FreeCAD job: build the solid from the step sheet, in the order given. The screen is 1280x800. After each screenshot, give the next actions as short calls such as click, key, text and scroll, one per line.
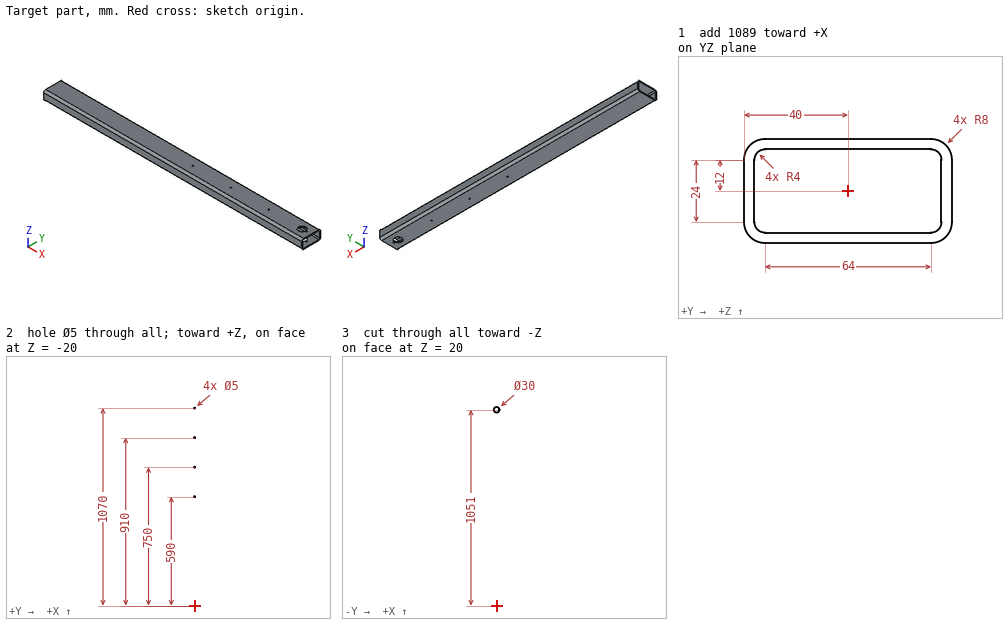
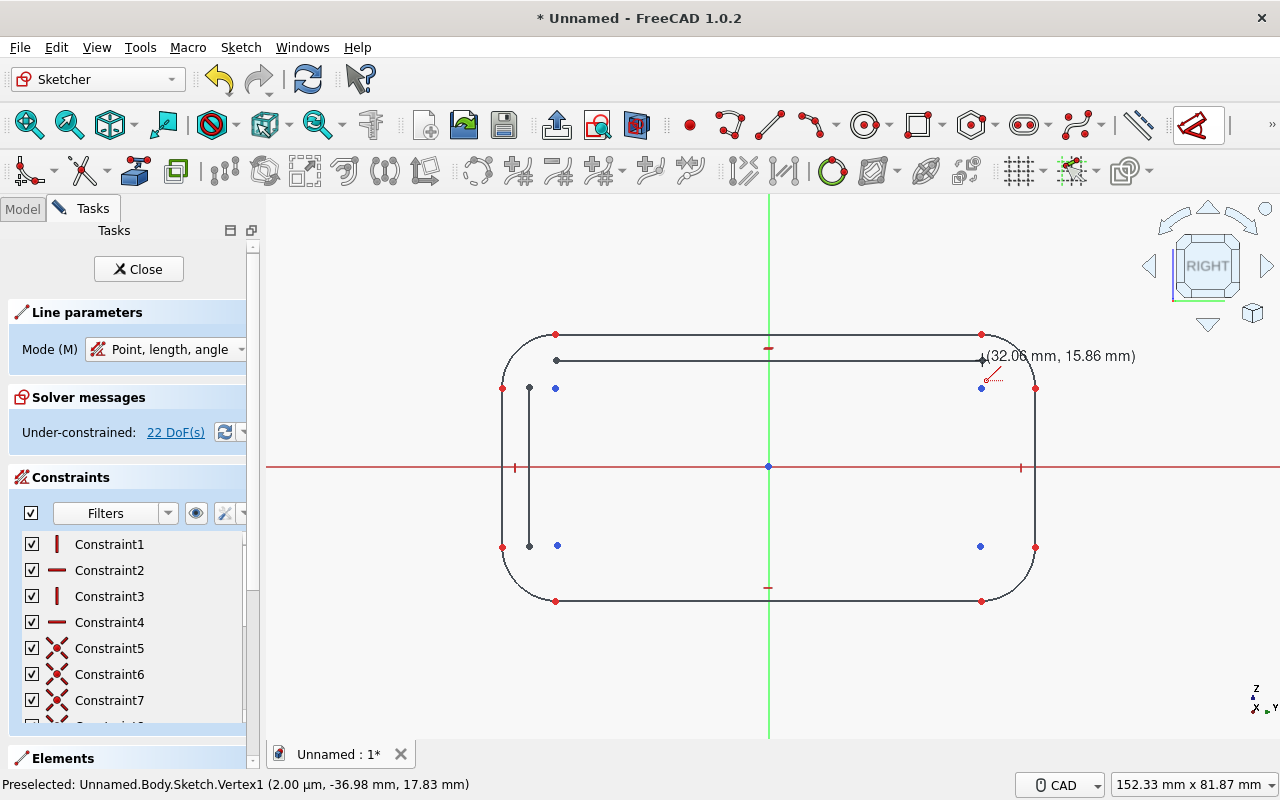
click(1008, 387)
click(1008, 546)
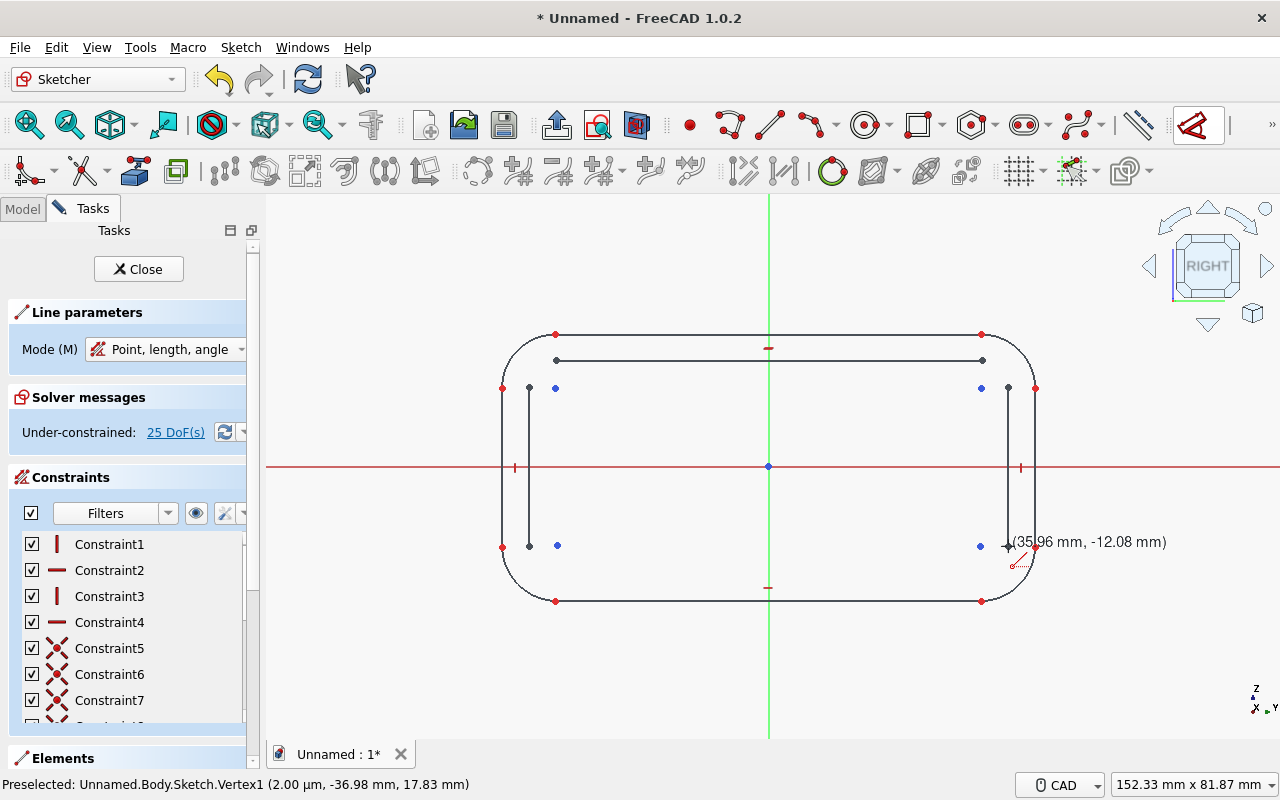
click(982, 573)
click(556, 573)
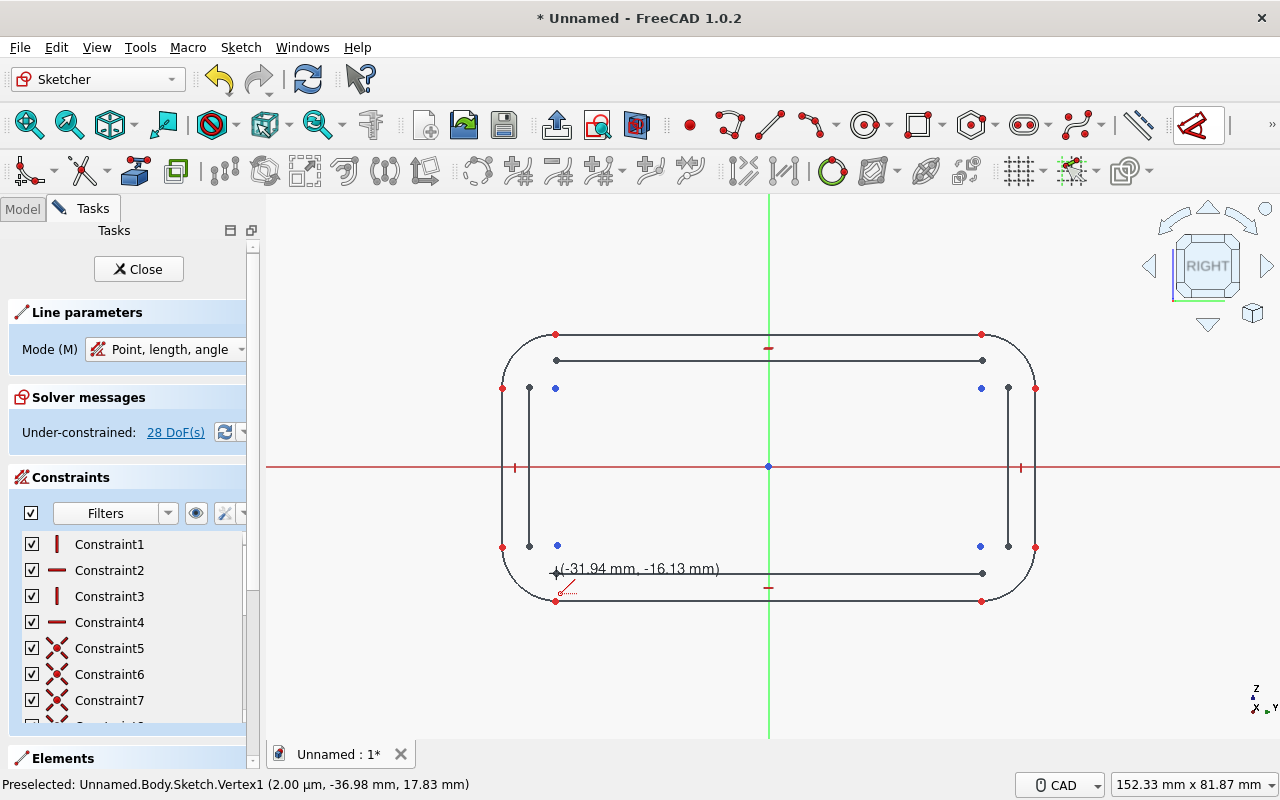
click(812, 126)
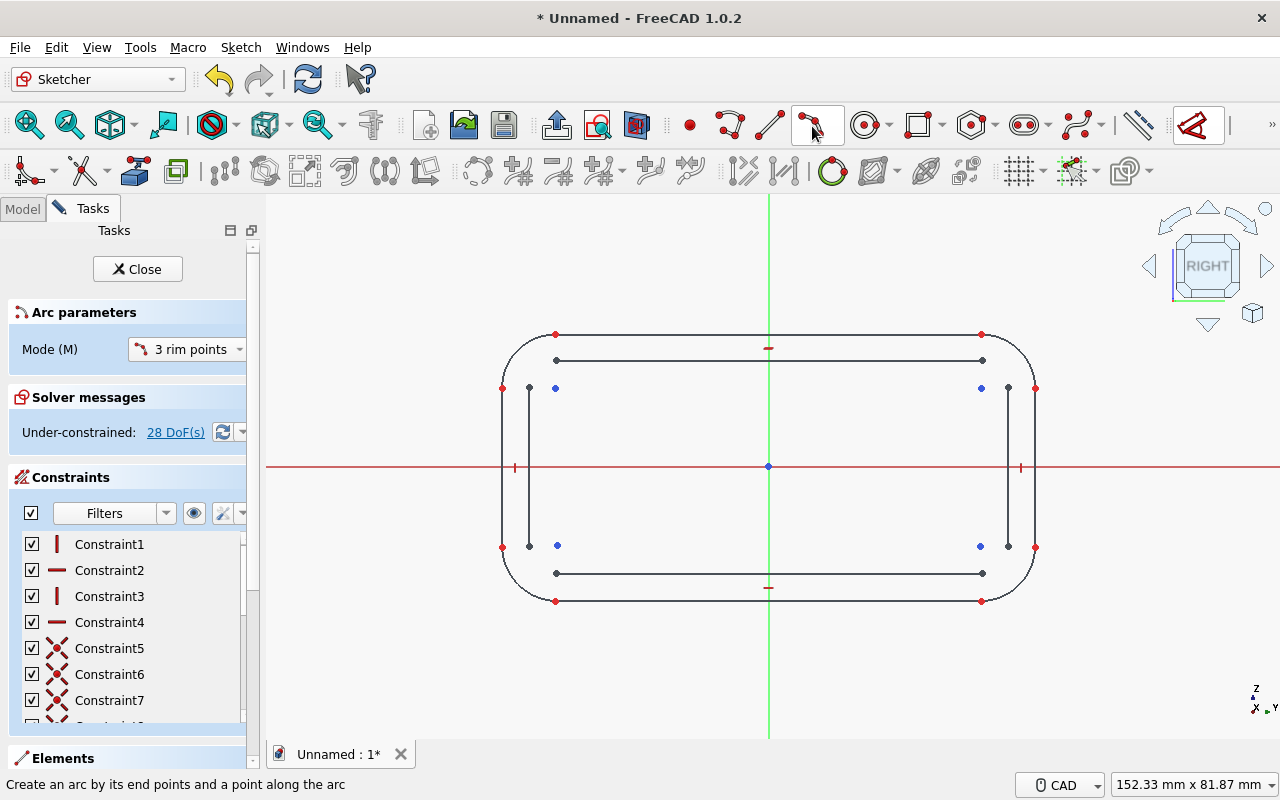
click(529, 388)
click(556, 361)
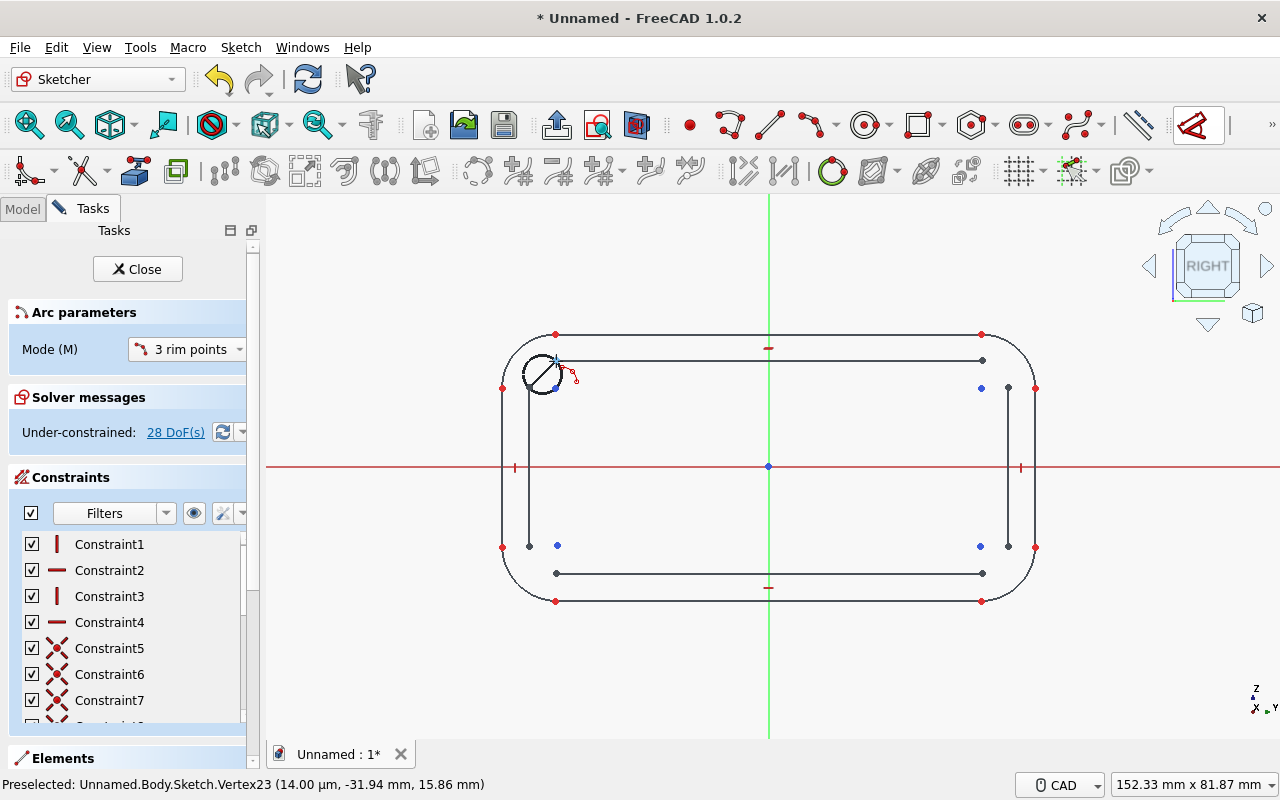
scroll(537, 368, up, 4)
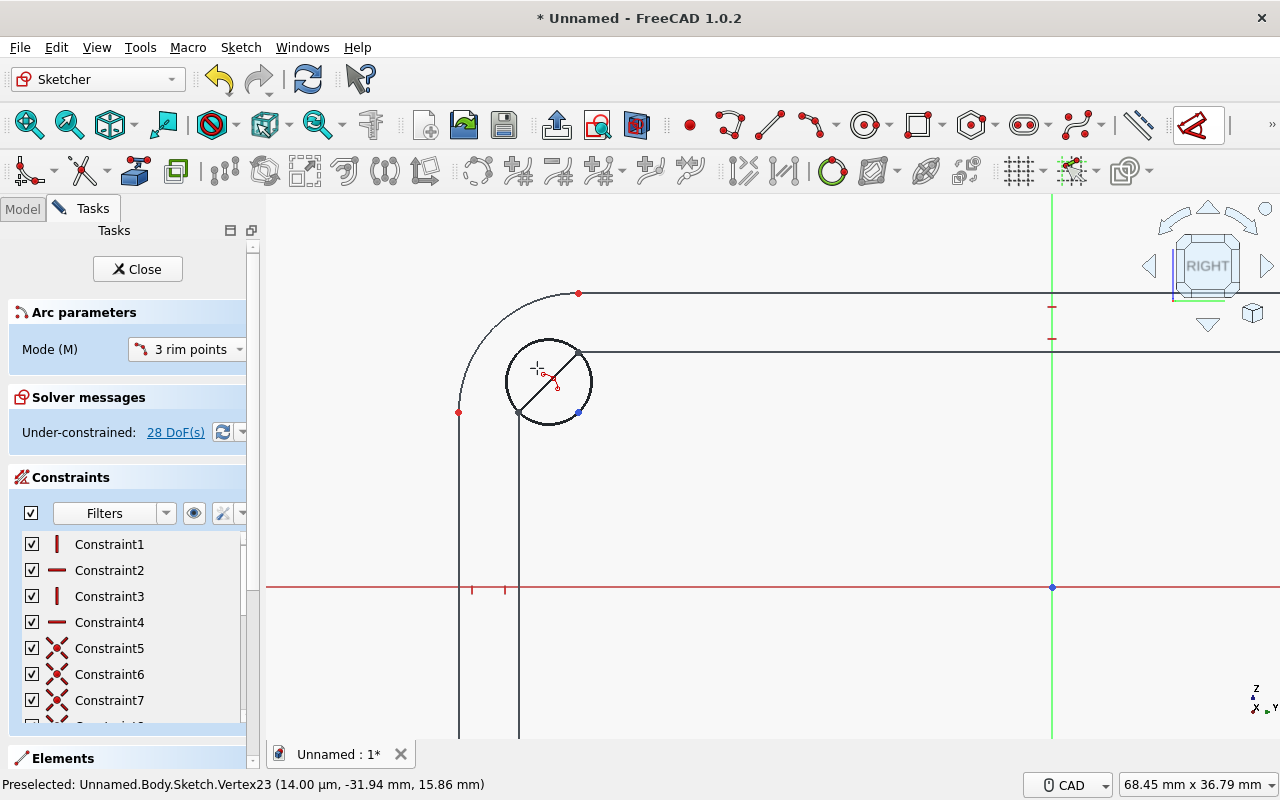
click(536, 367)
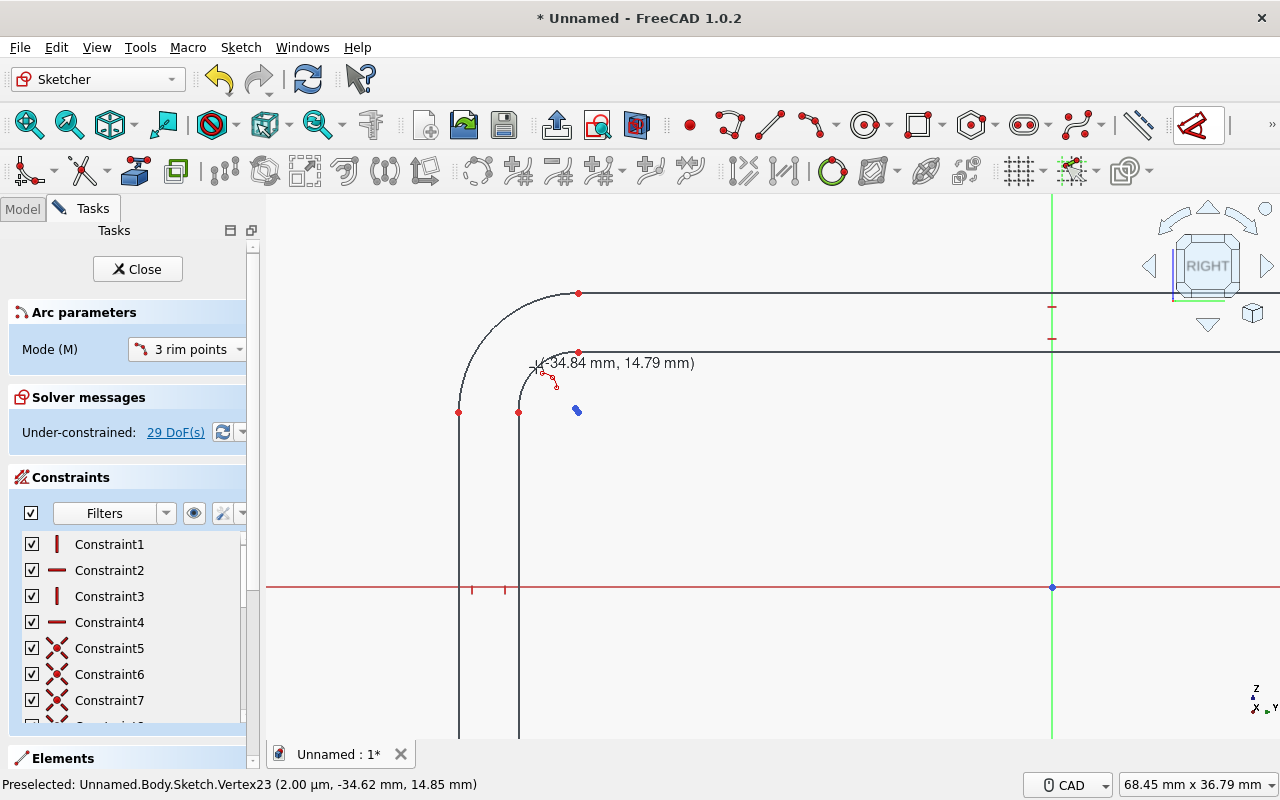
scroll(421, 368, down, 4)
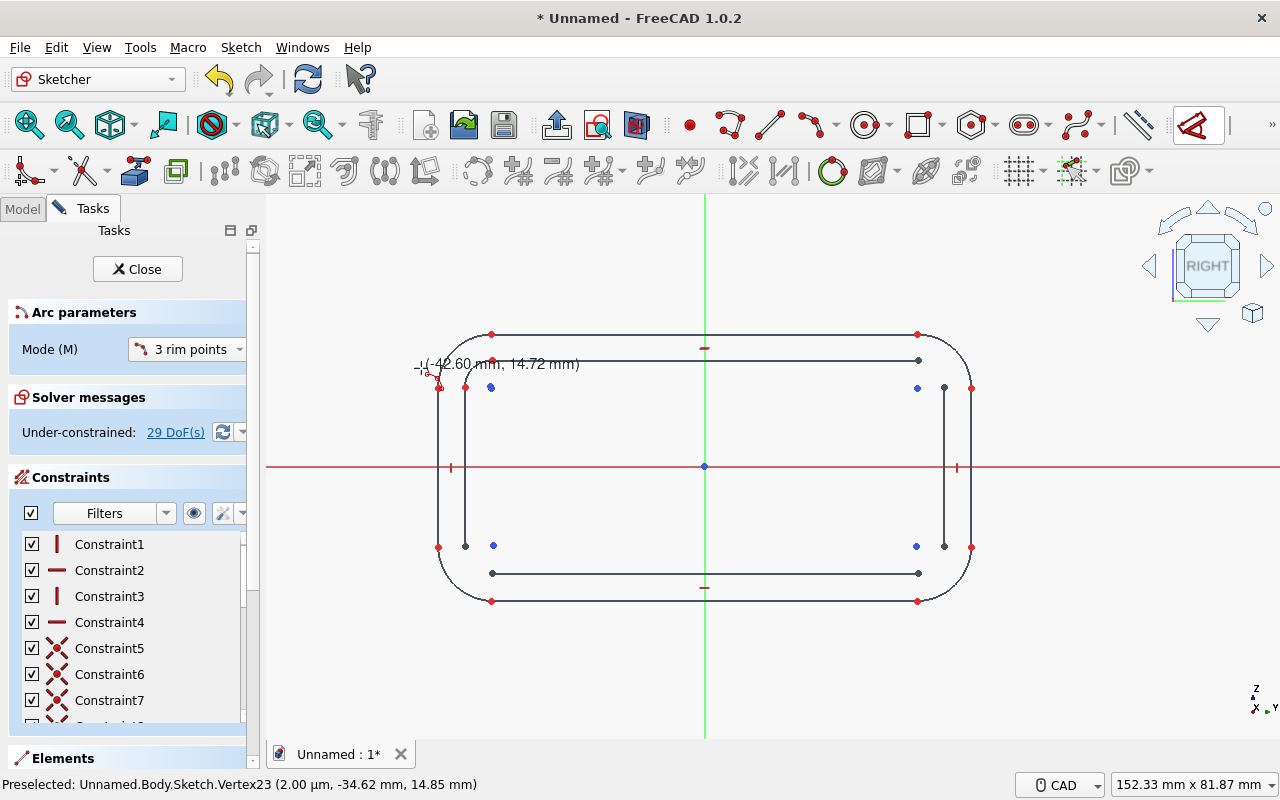
click(918, 361)
click(944, 388)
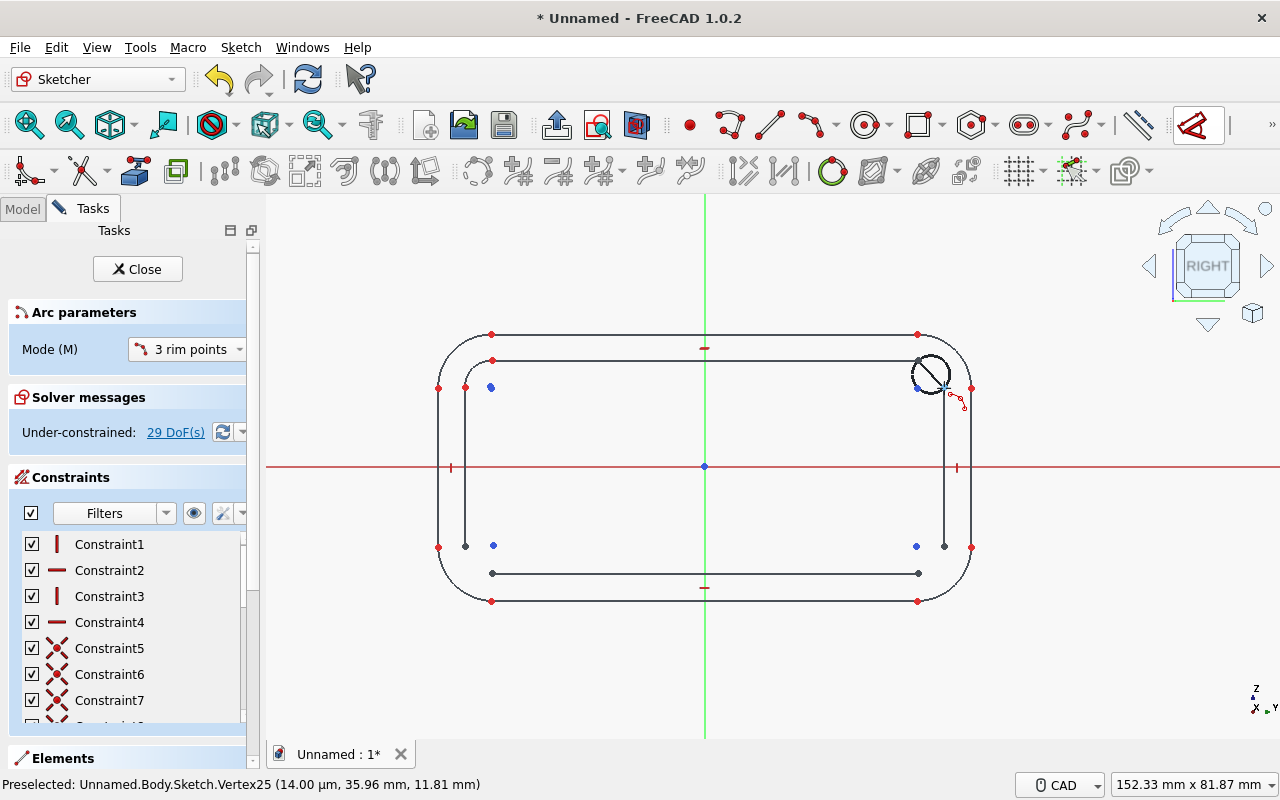
scroll(937, 368, up, 4)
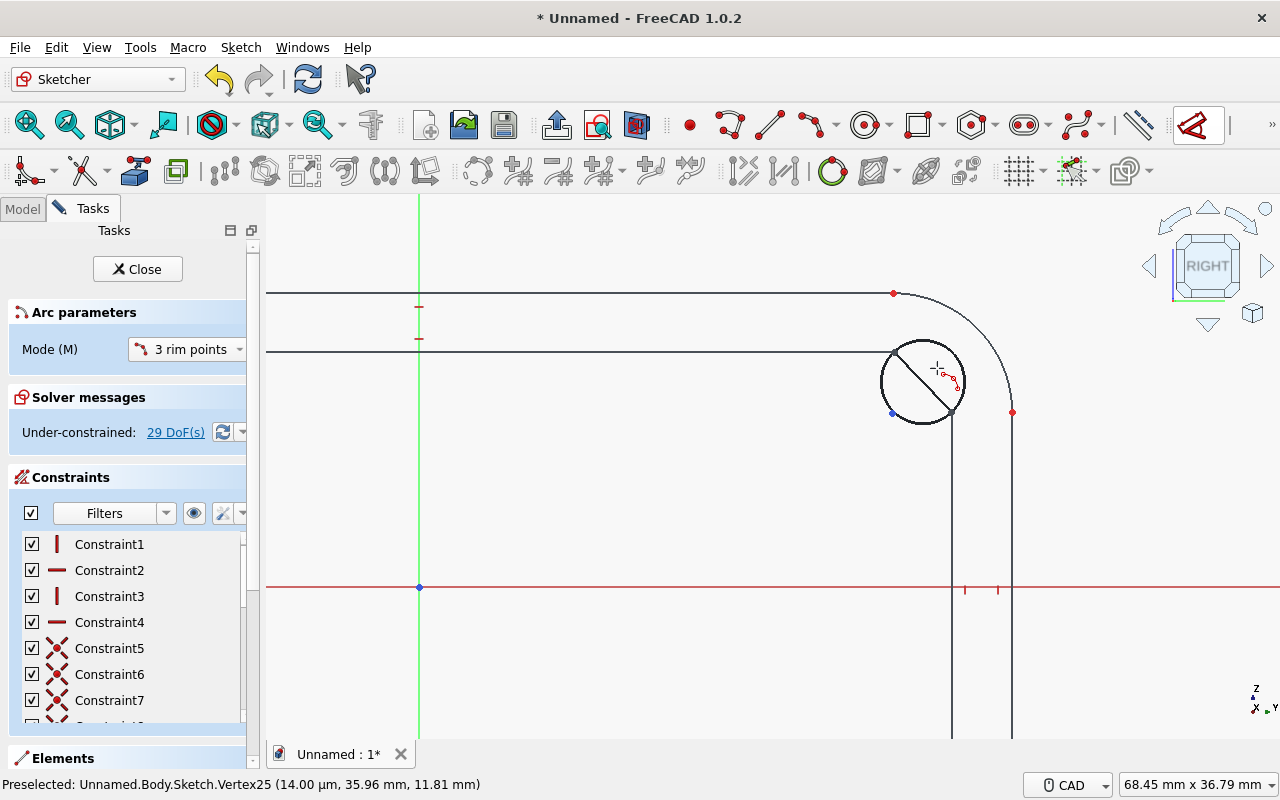
click(935, 367)